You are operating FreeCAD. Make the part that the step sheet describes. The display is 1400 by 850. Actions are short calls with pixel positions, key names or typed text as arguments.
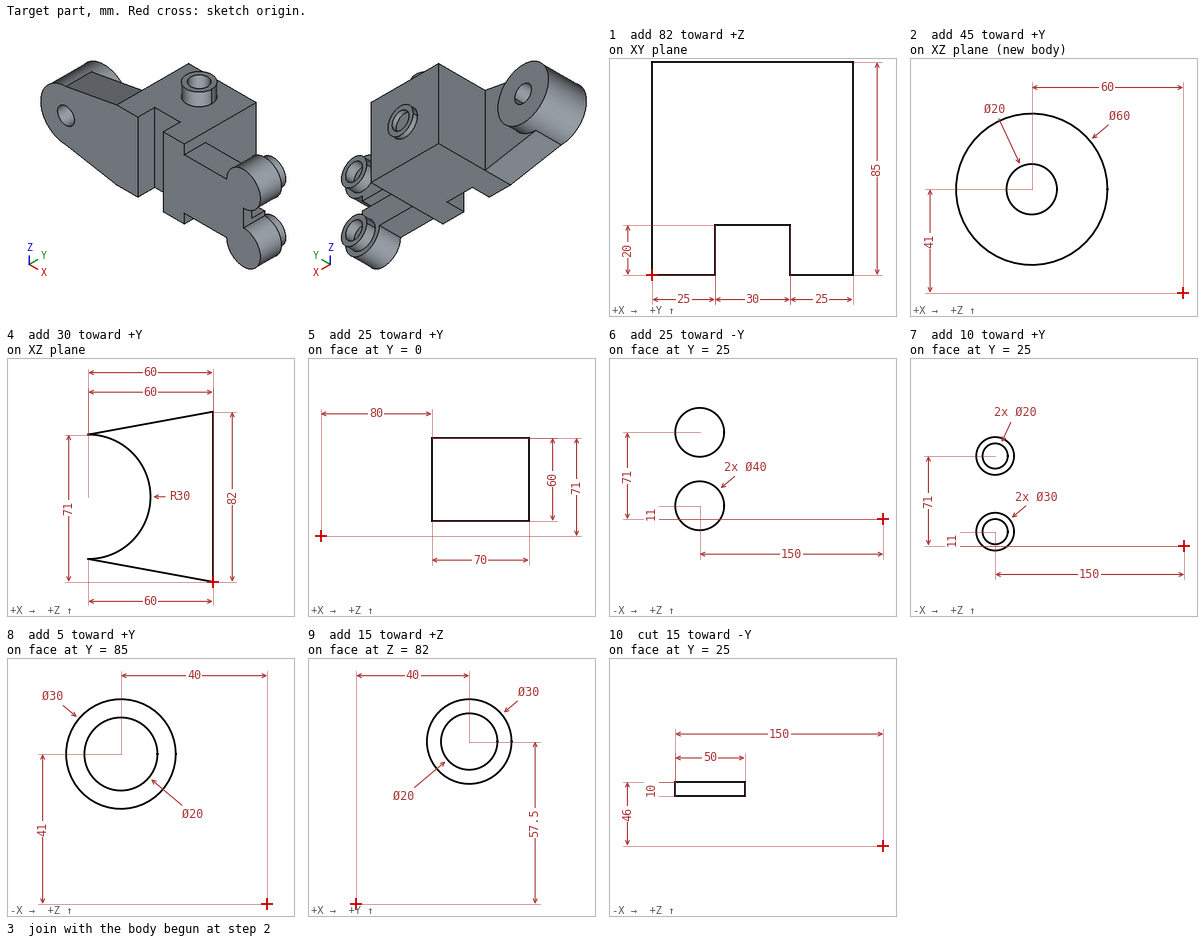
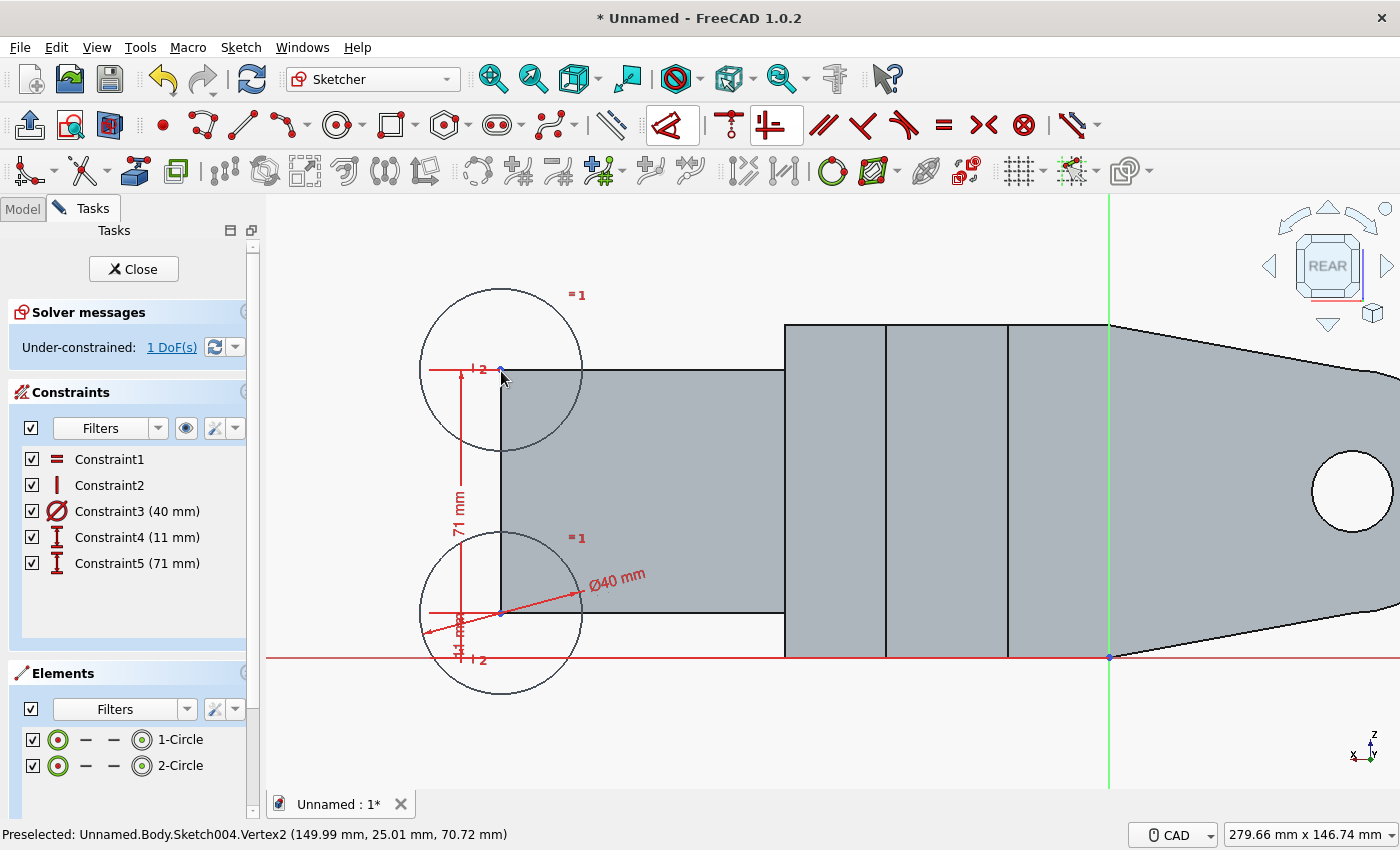
click(501, 613)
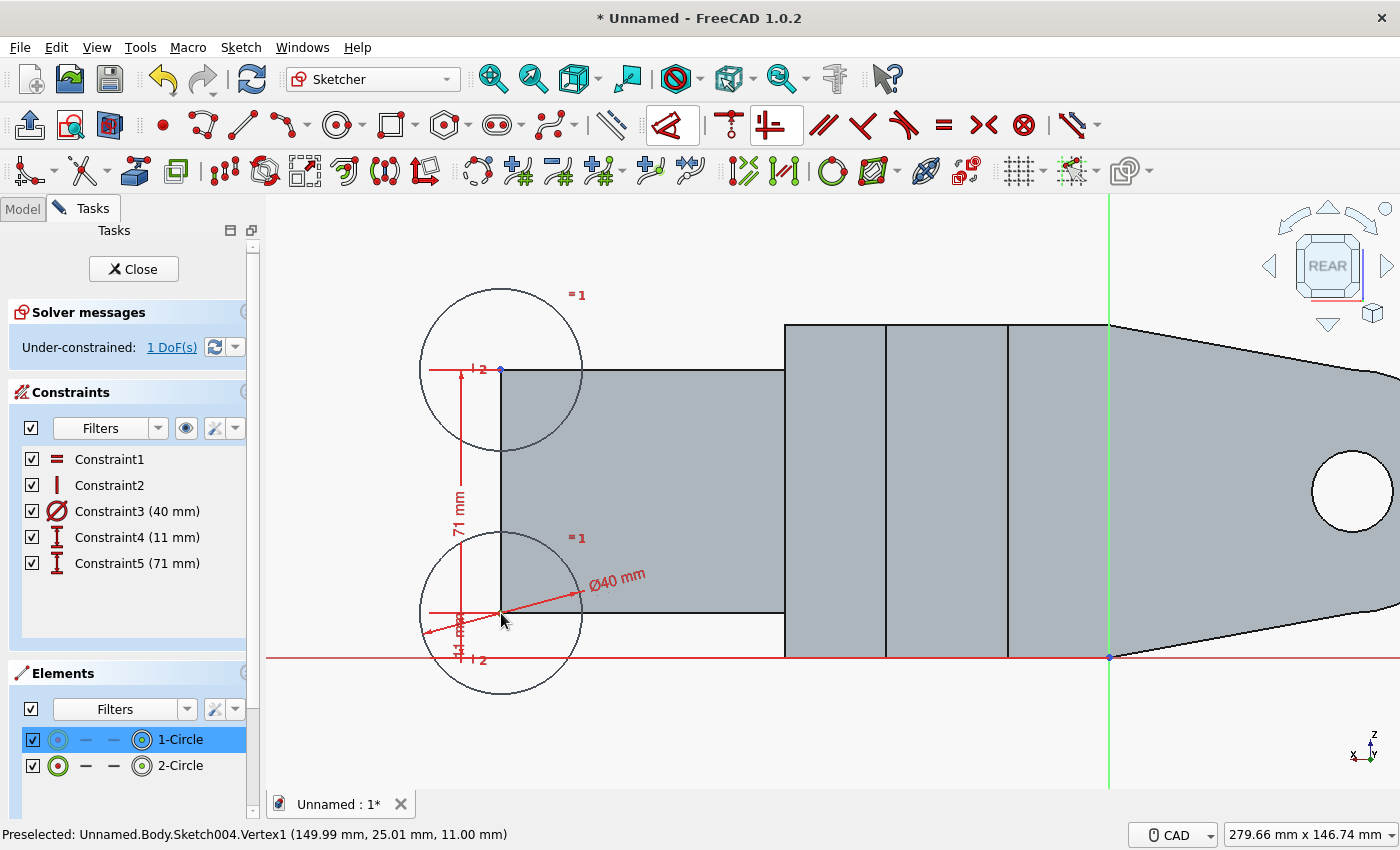
key(l)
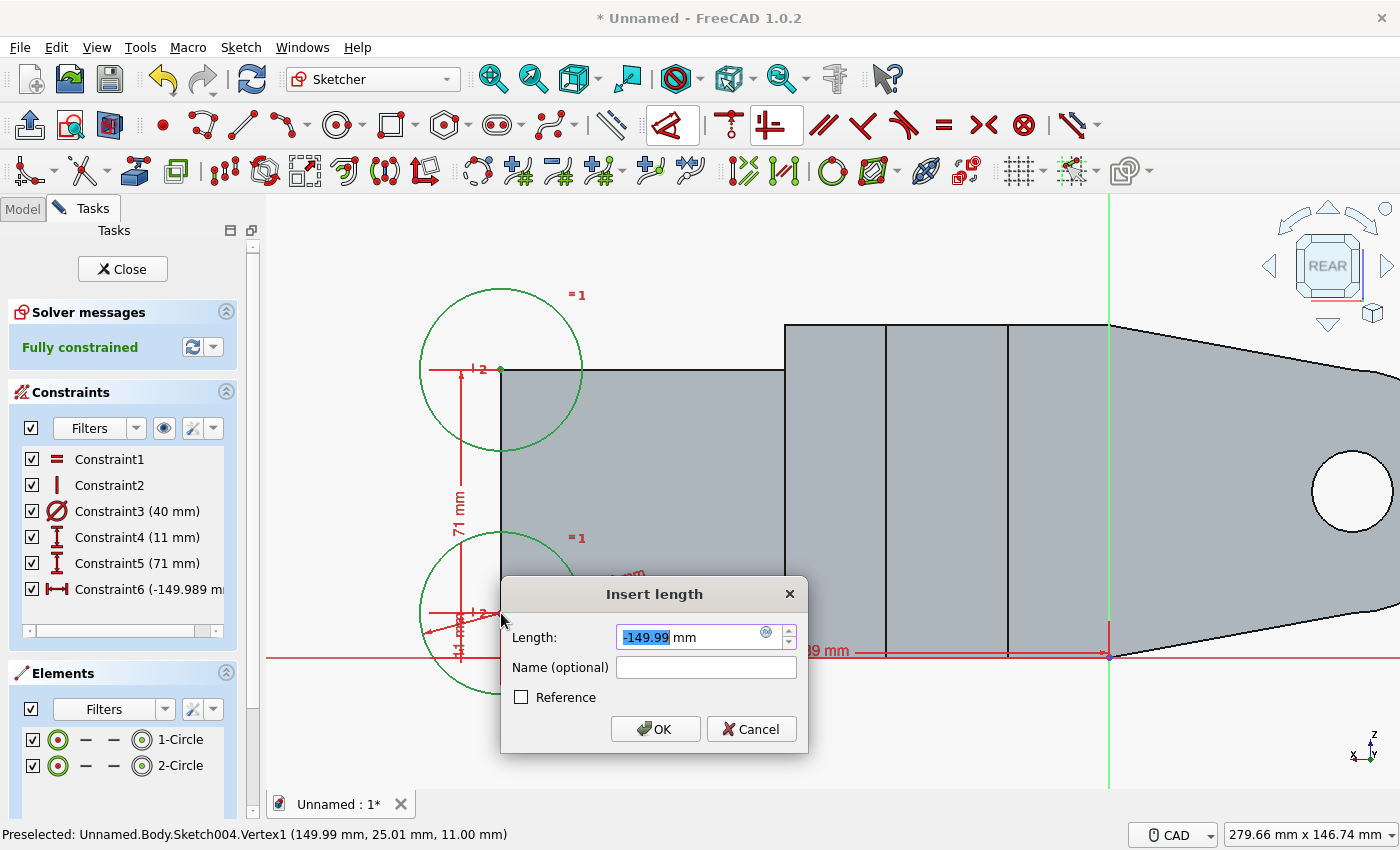
text(-150)
key(Return)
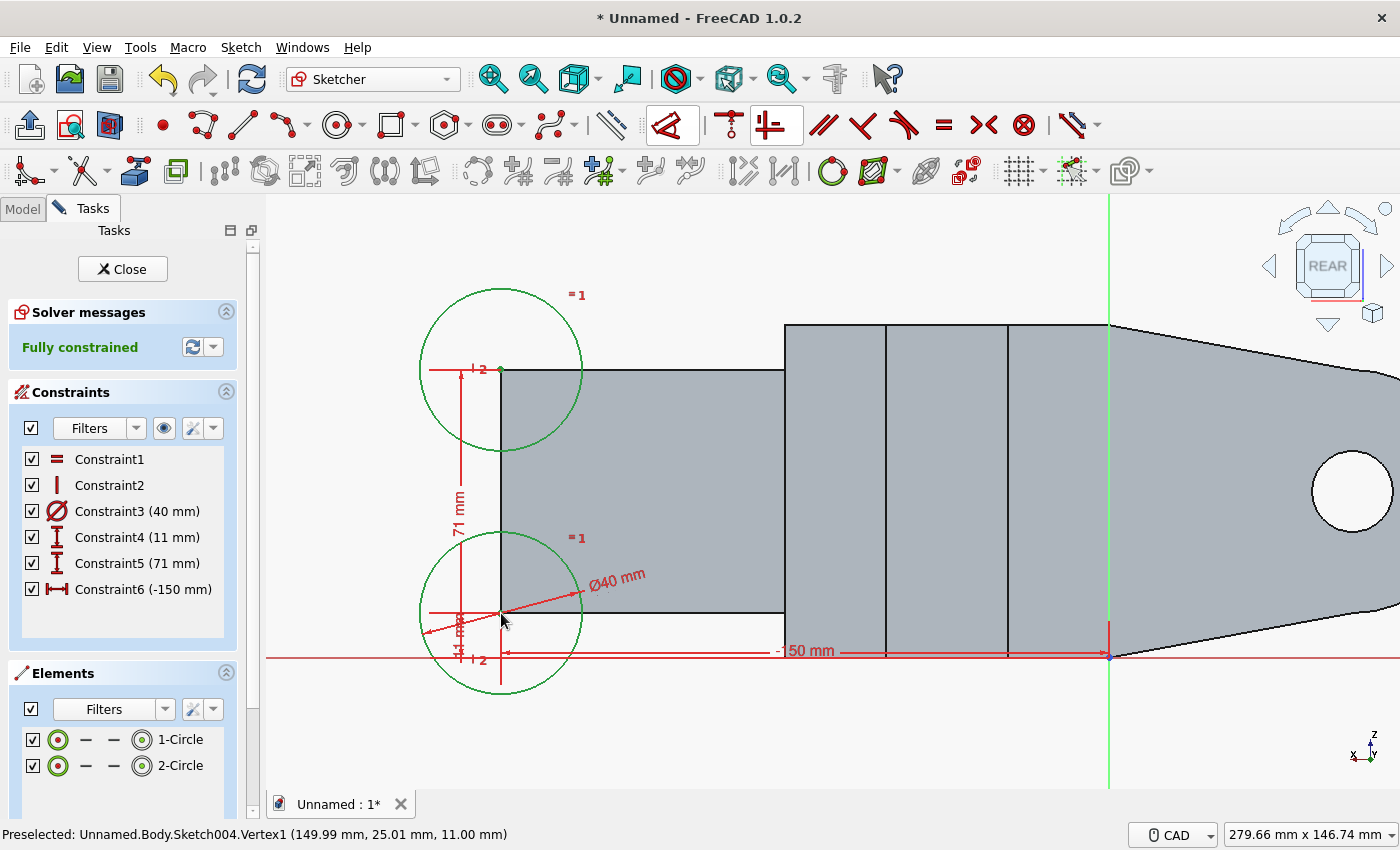
click(123, 269)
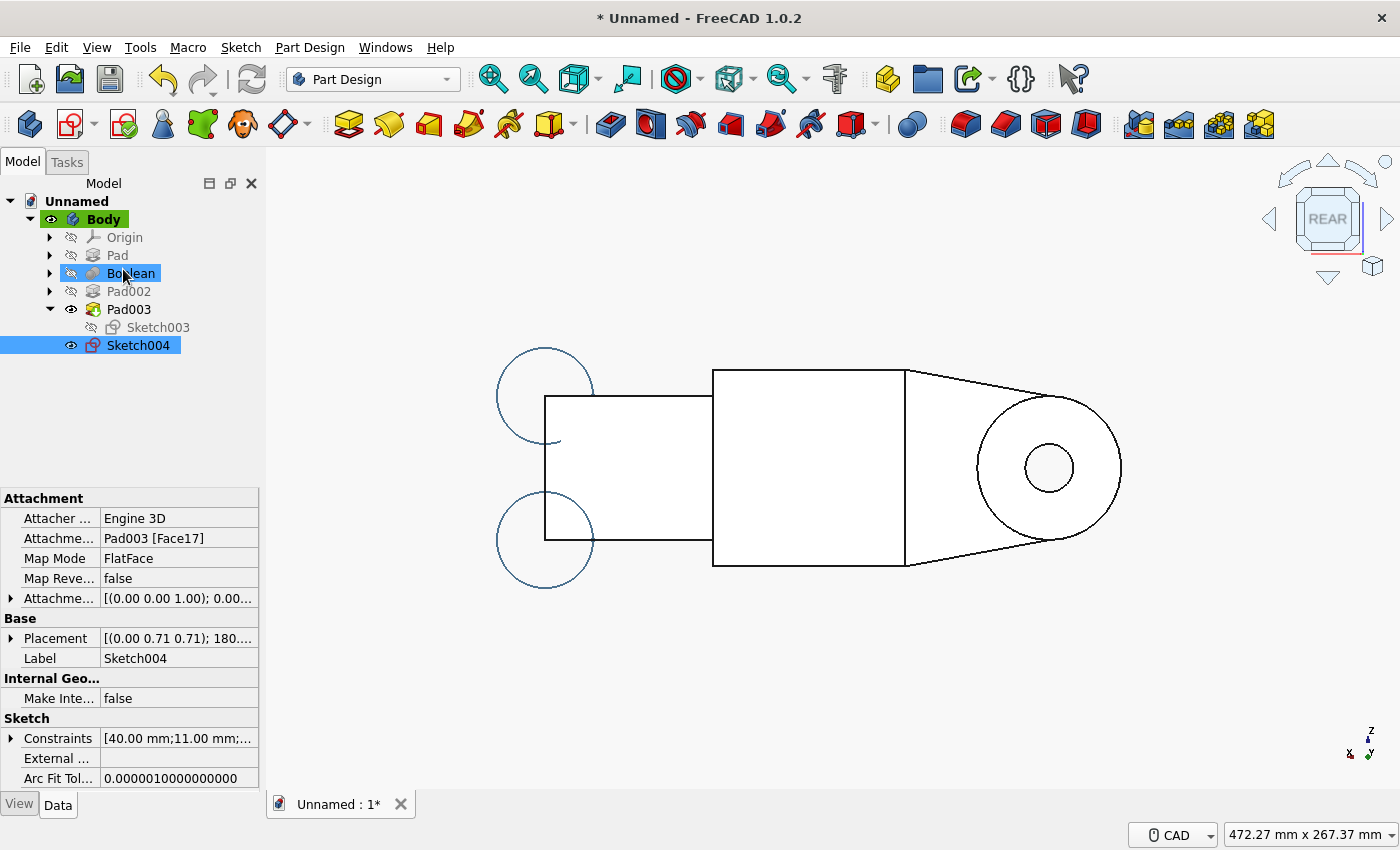
click(350, 124)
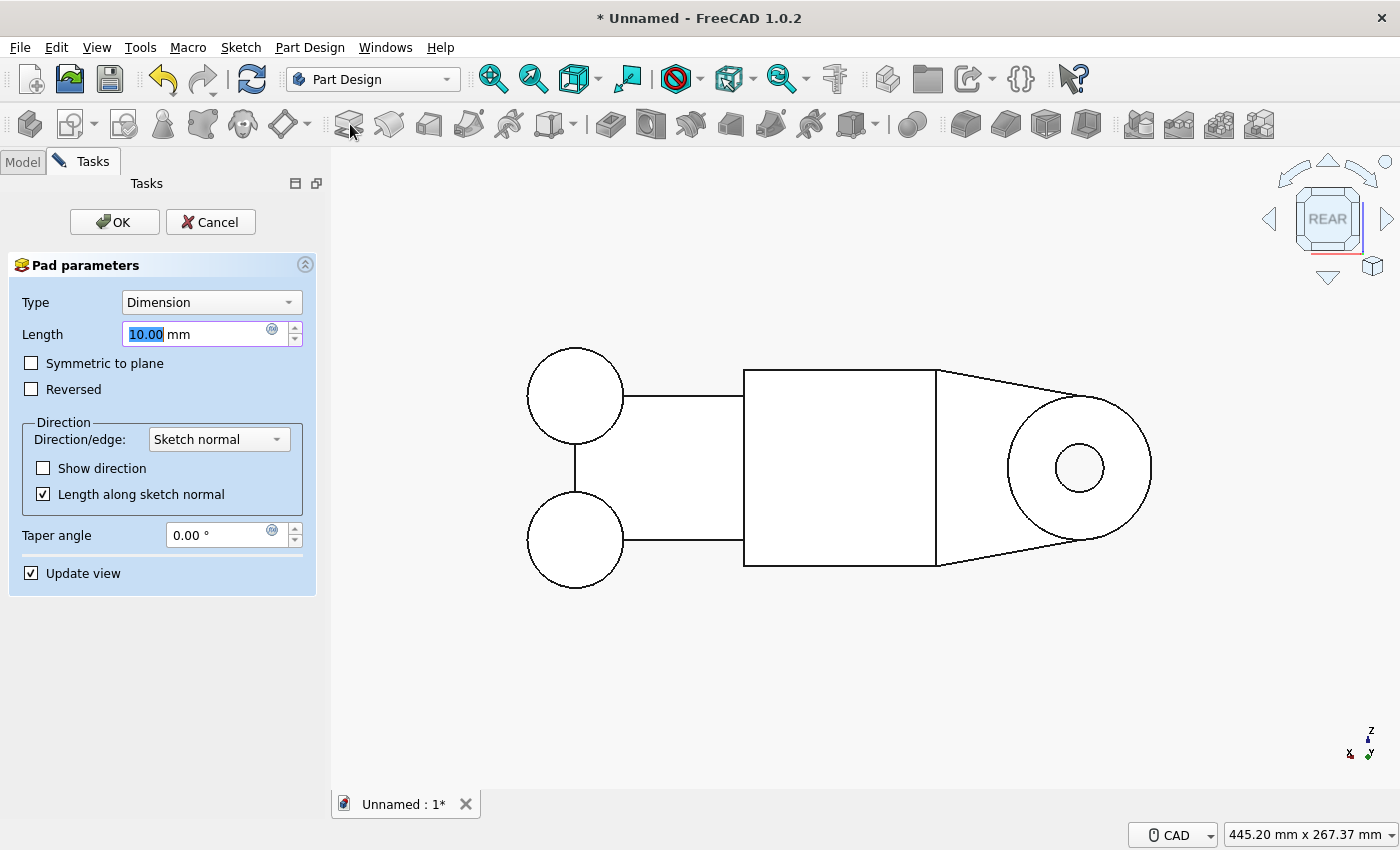
text(25)
key(Tab)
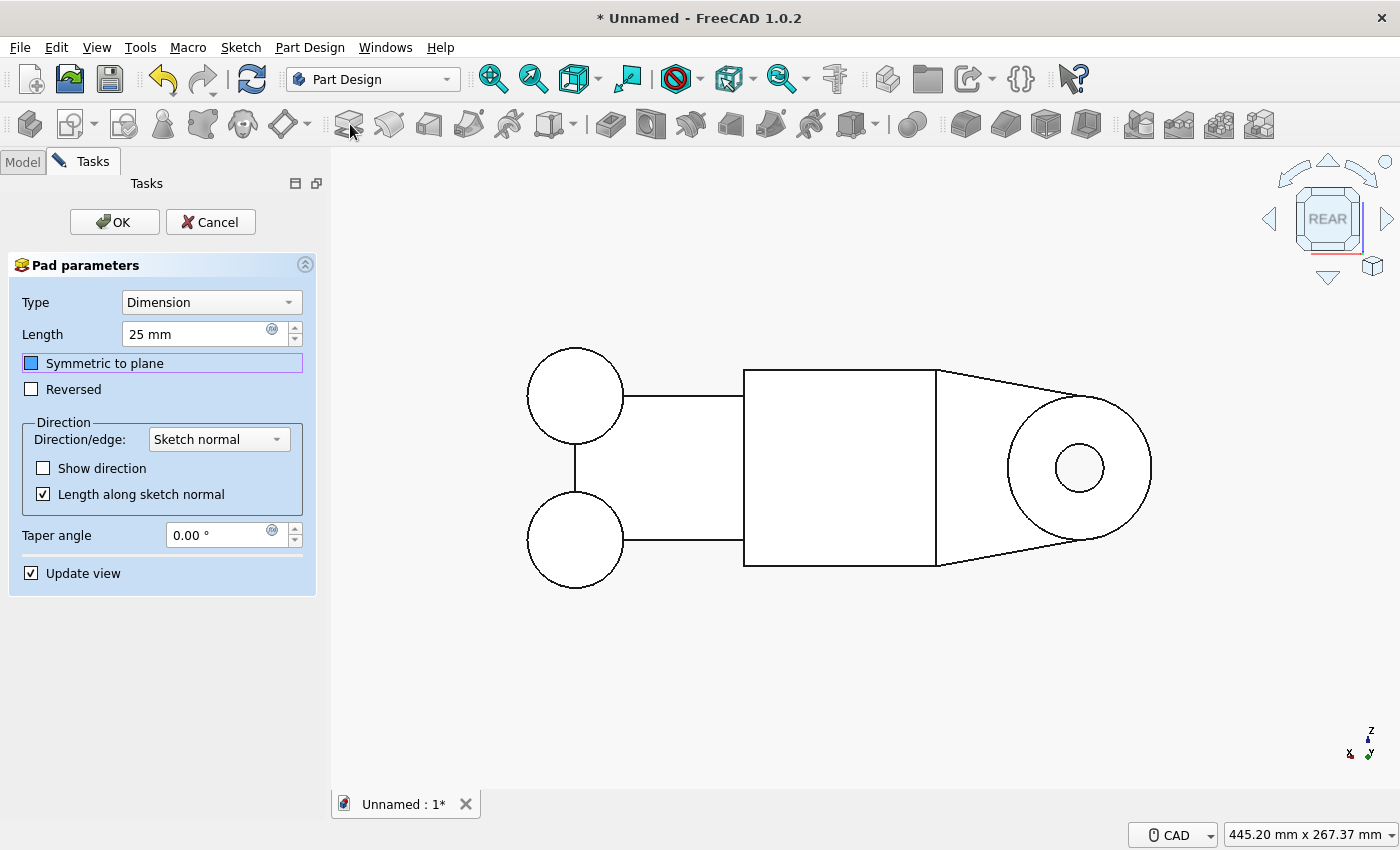
click(30, 389)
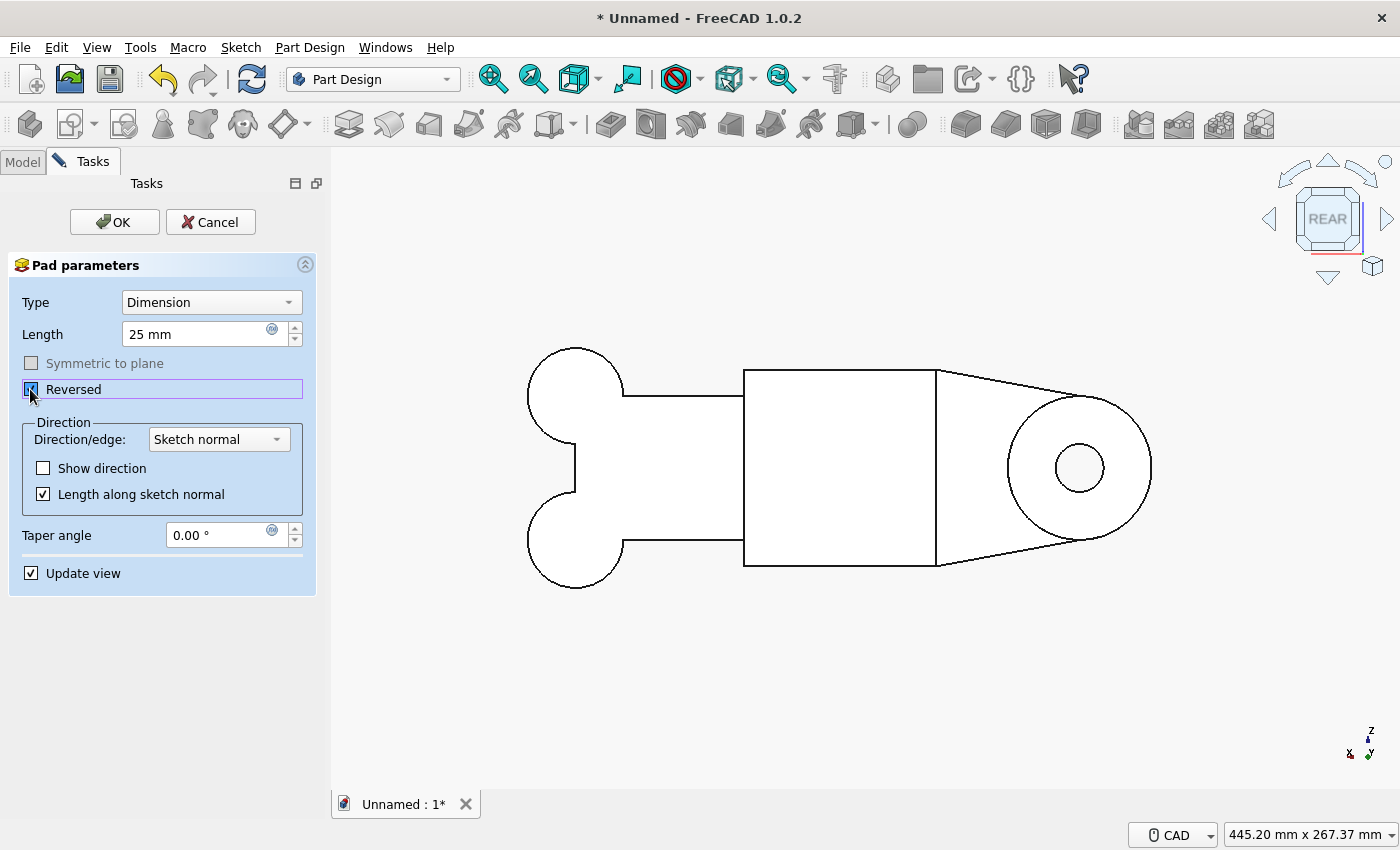
click(115, 222)